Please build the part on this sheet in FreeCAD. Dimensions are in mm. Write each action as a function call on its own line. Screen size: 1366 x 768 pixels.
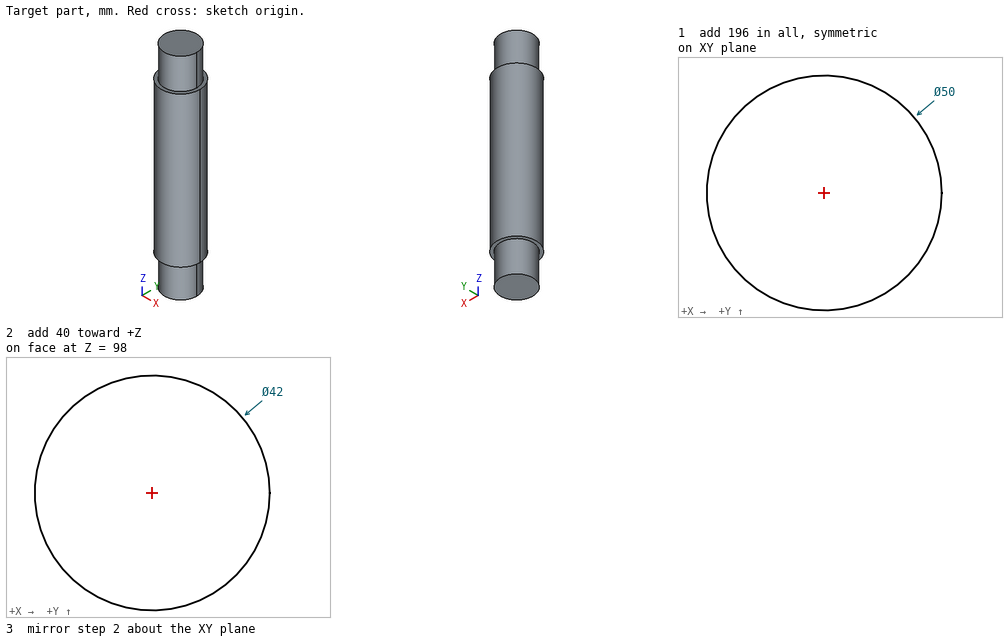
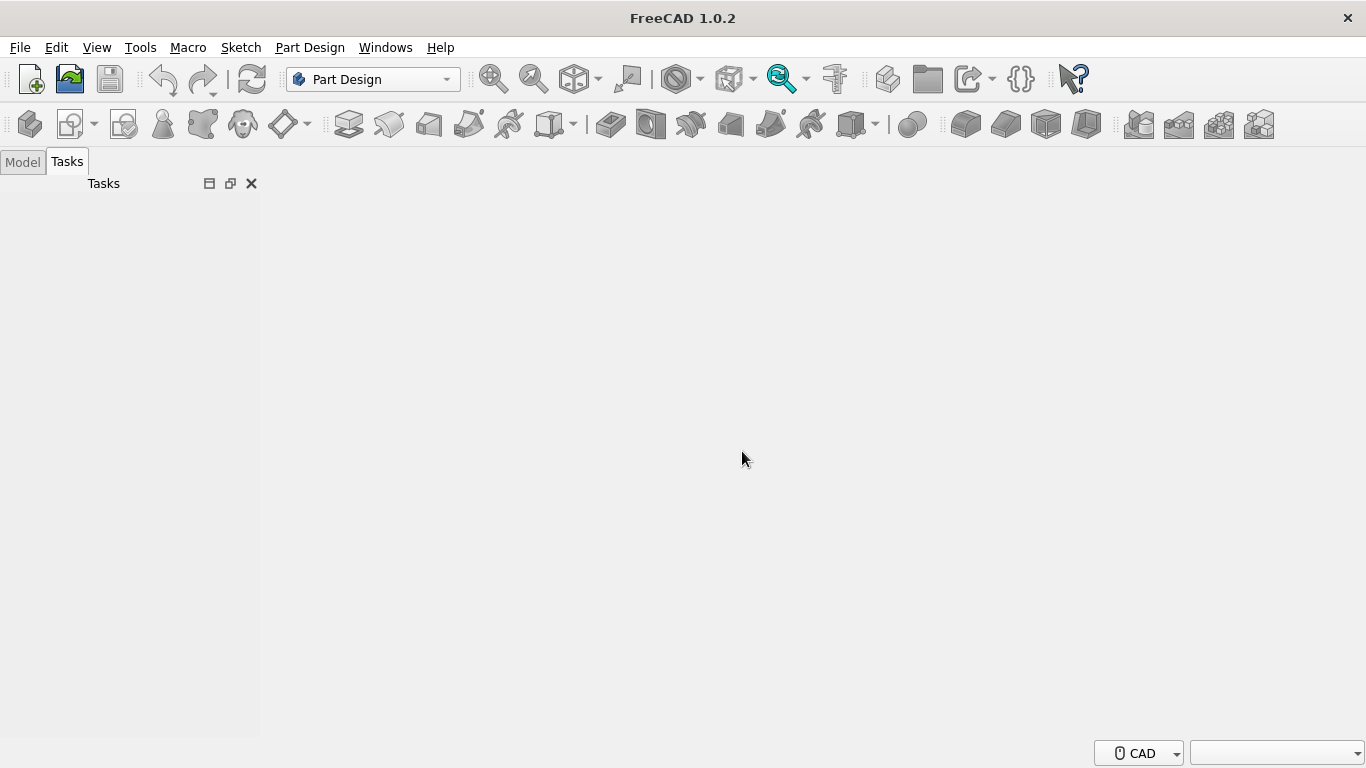
click(30, 80)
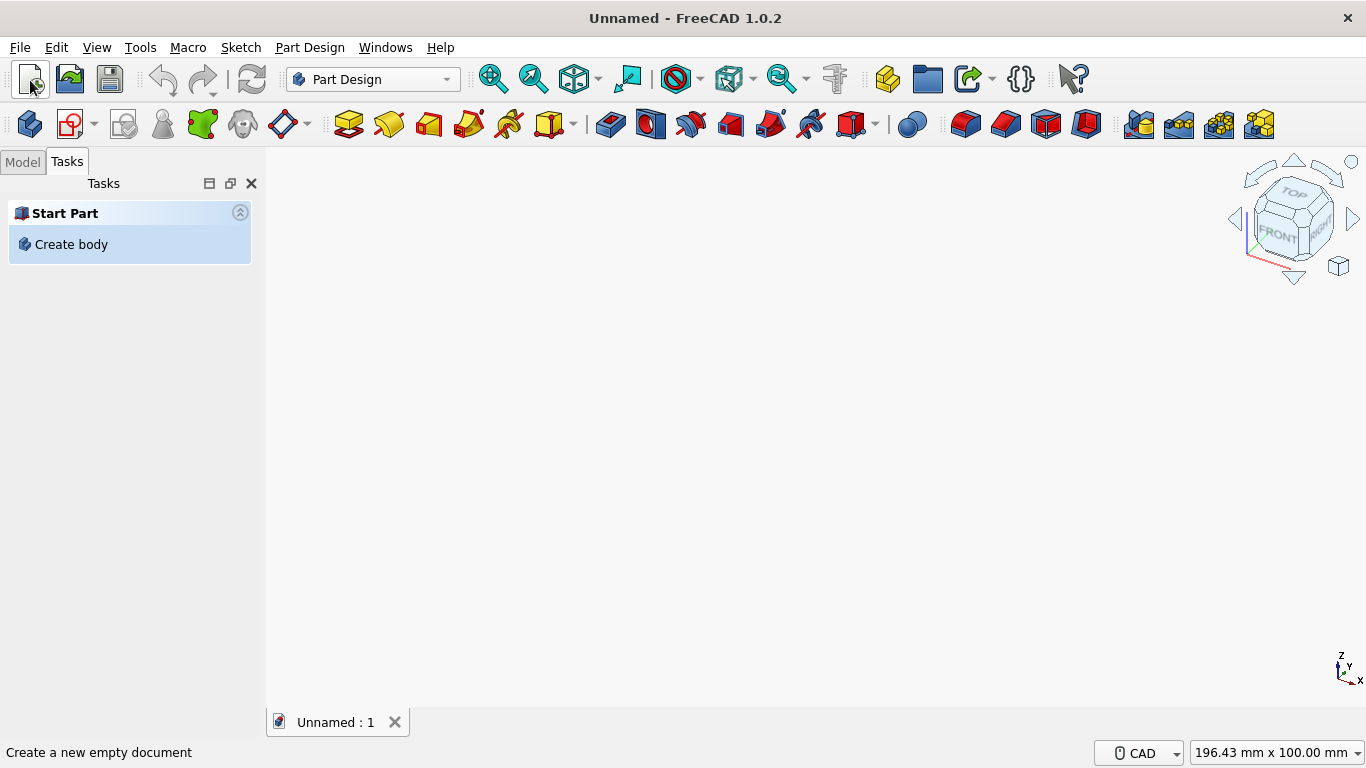
click(70, 124)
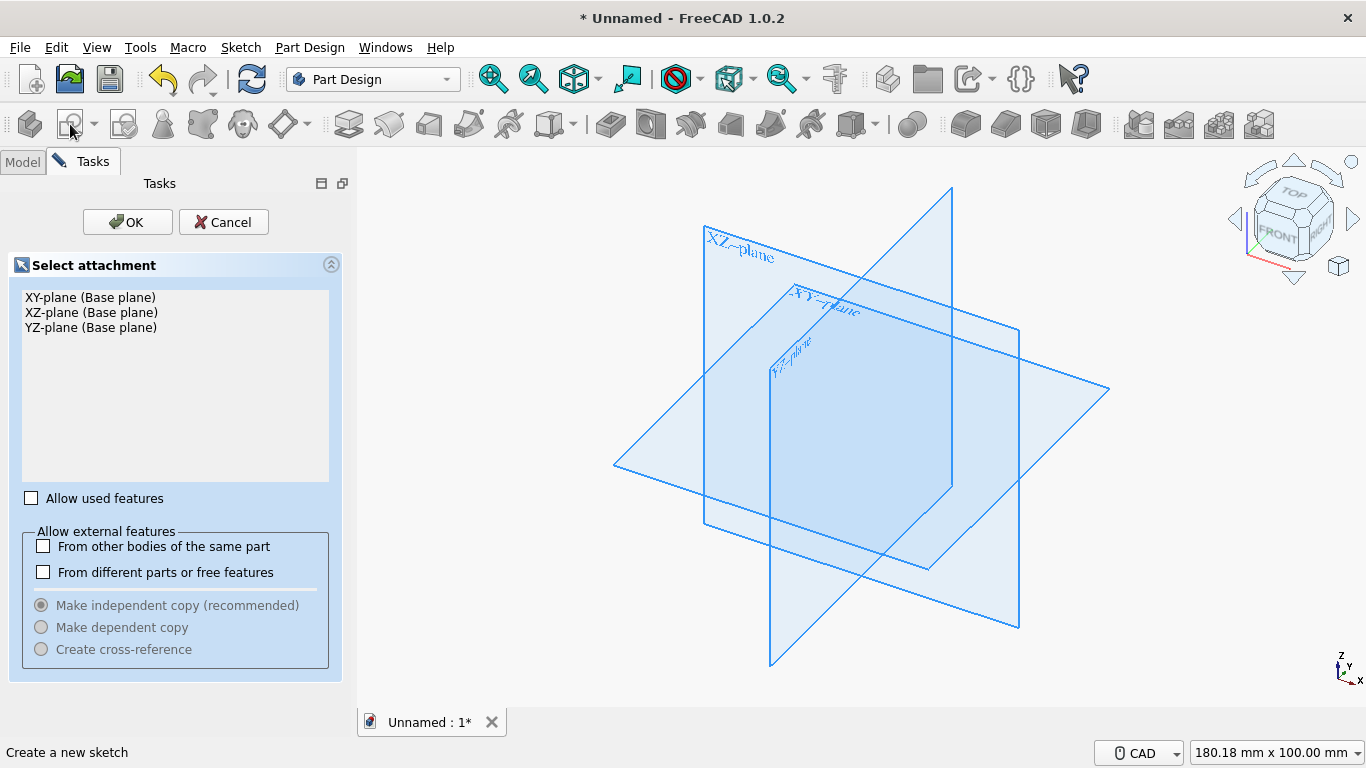
click(82, 298)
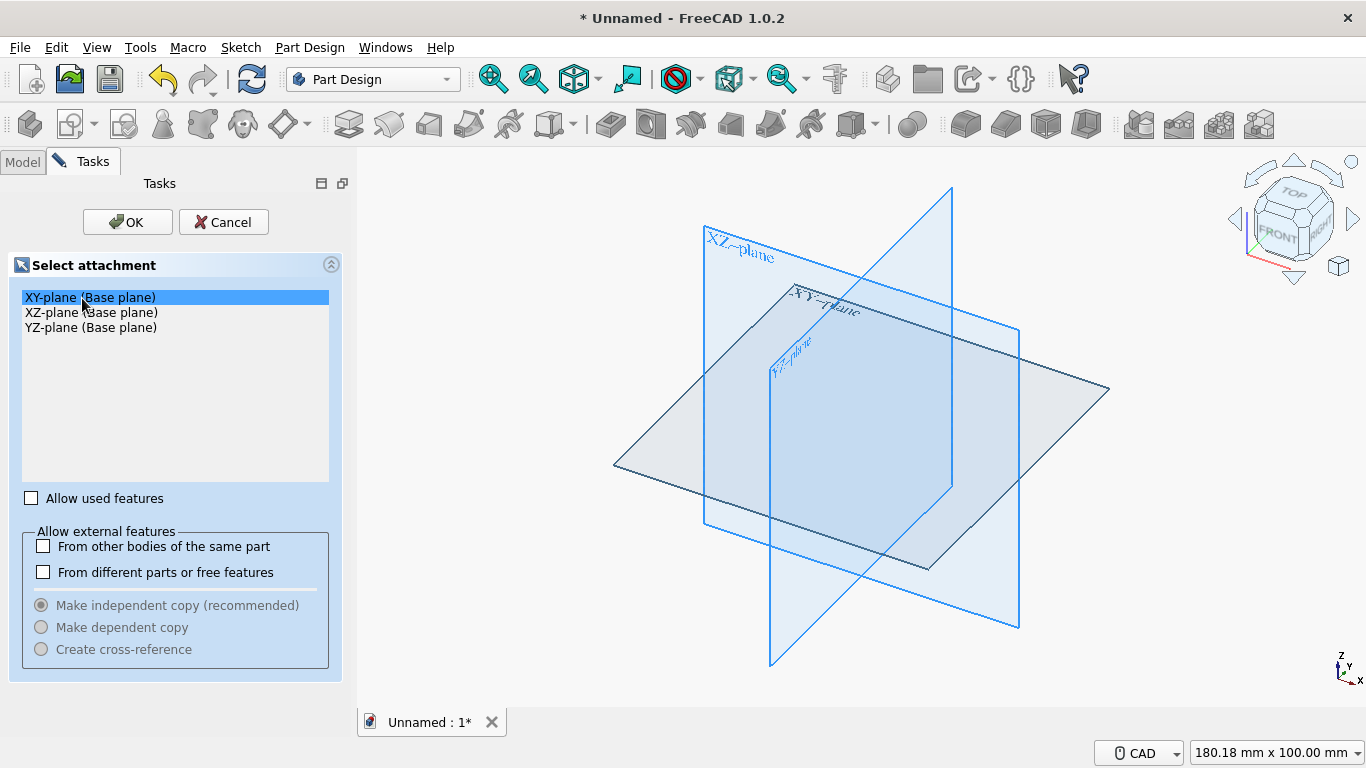
click(128, 222)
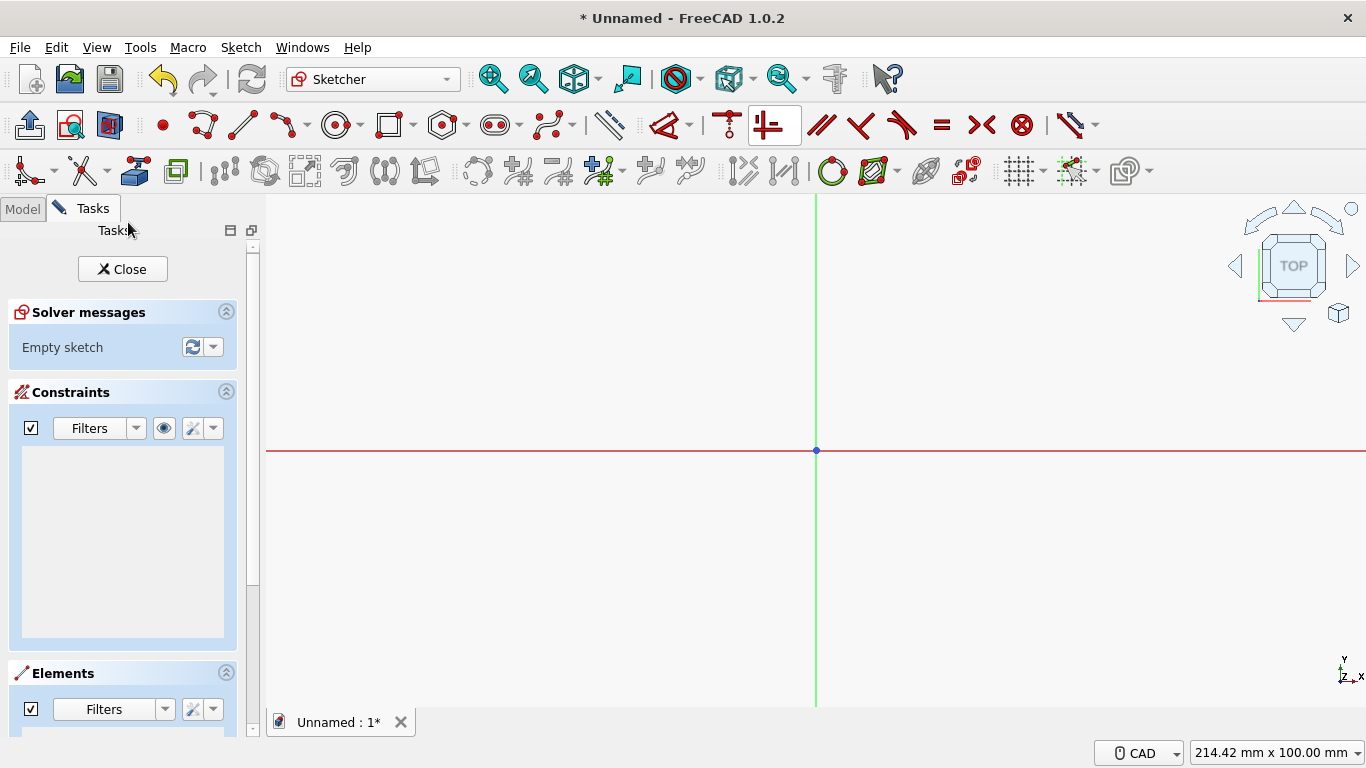
click(336, 126)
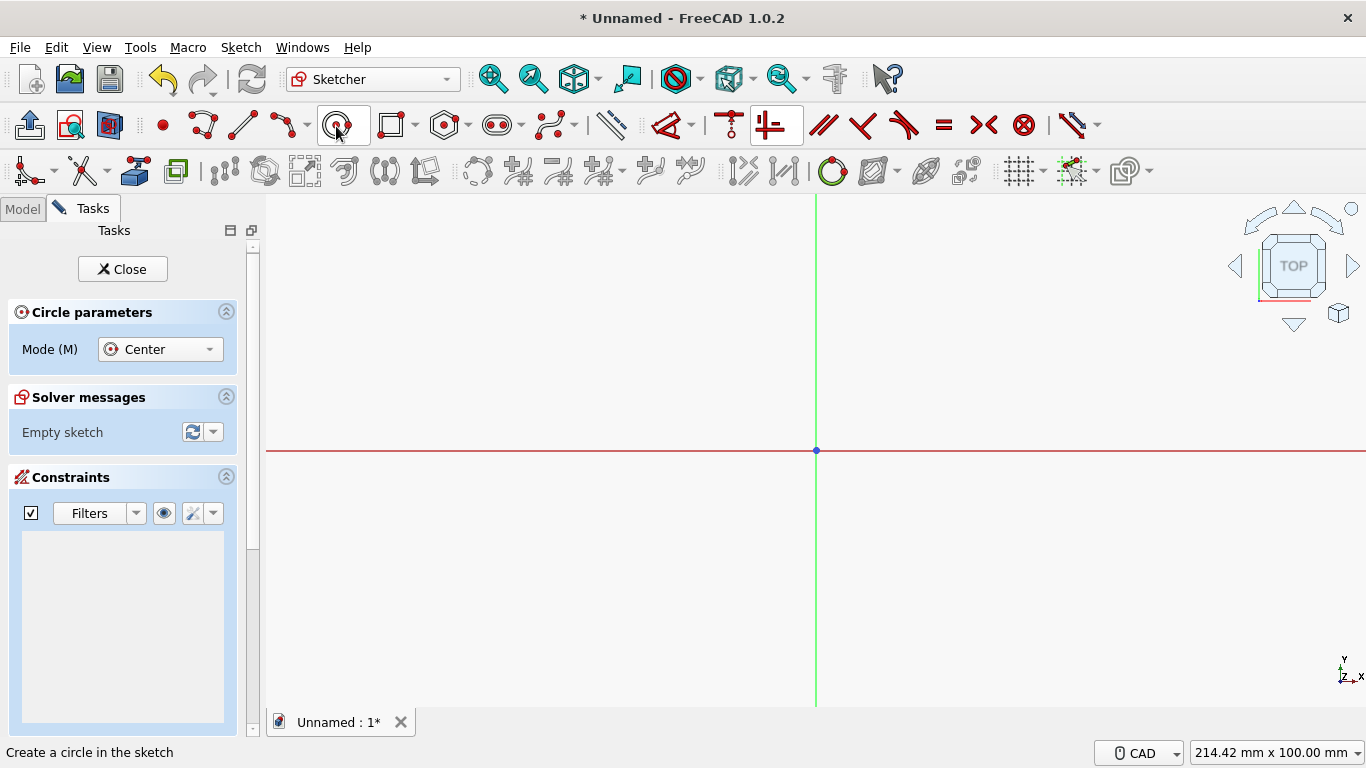
click(816, 450)
move(907, 360)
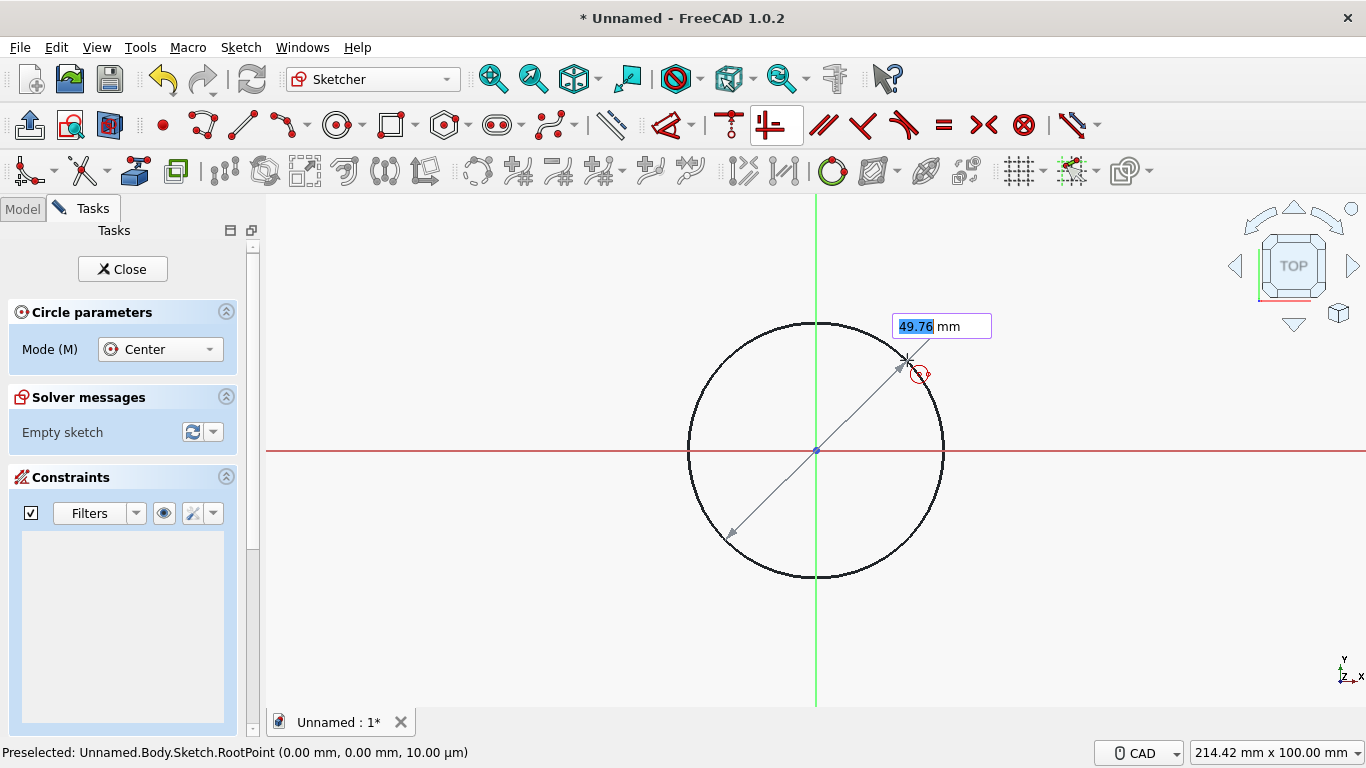
text(50)
key(Return)
key(Escape)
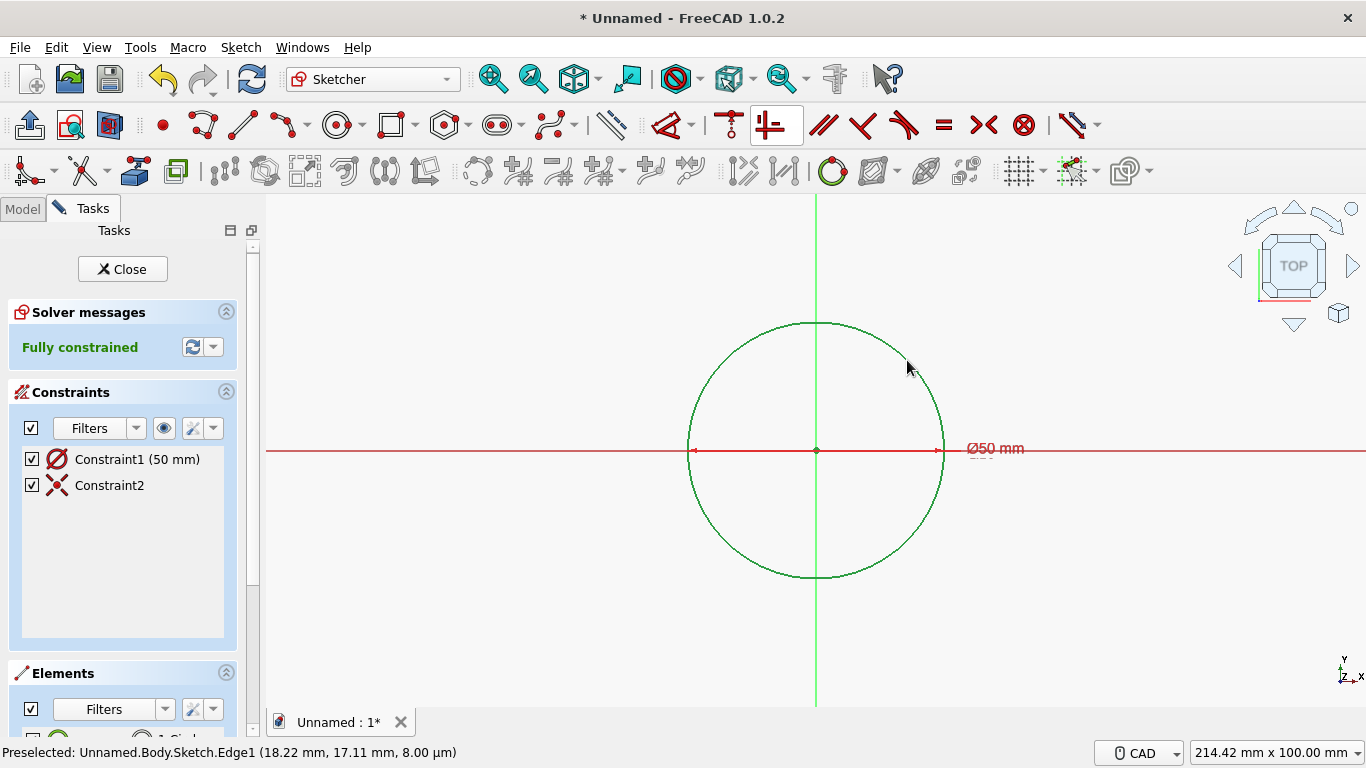
click(123, 269)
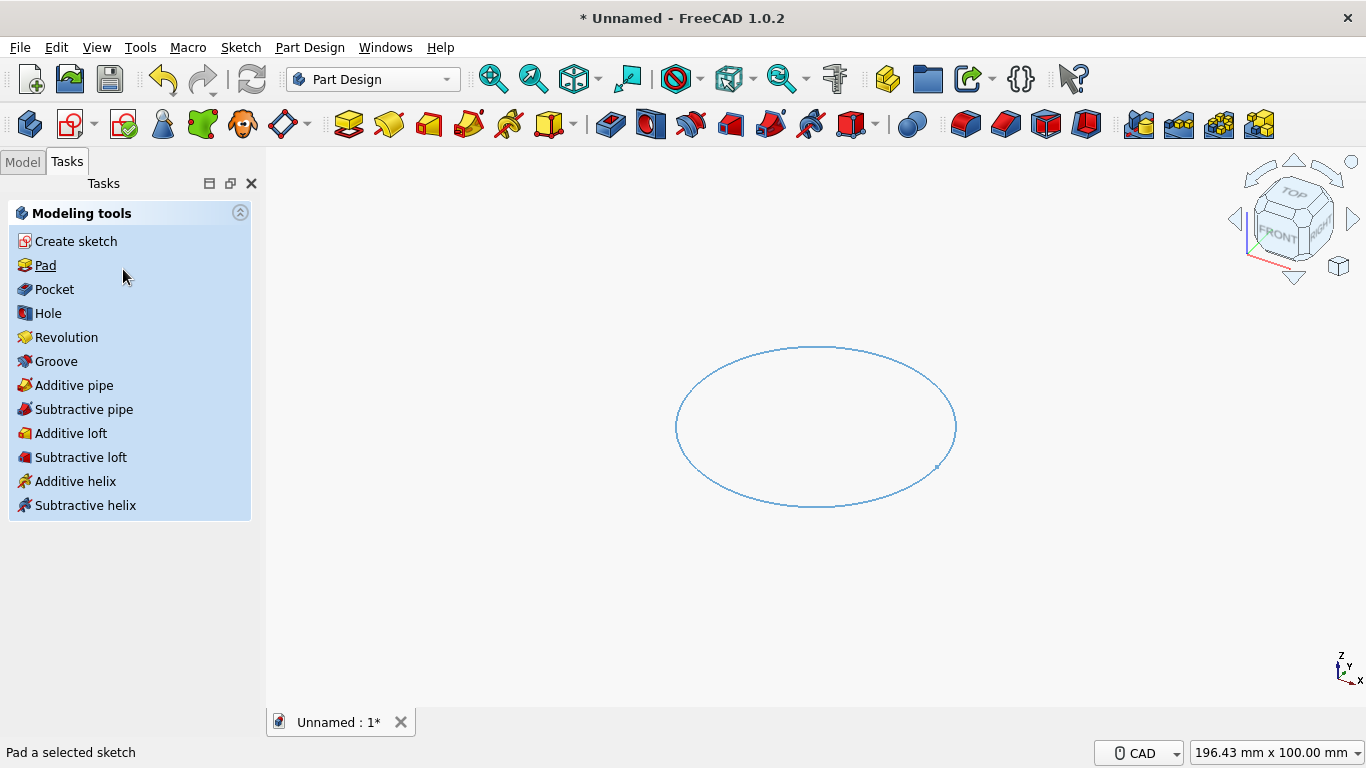
click(350, 124)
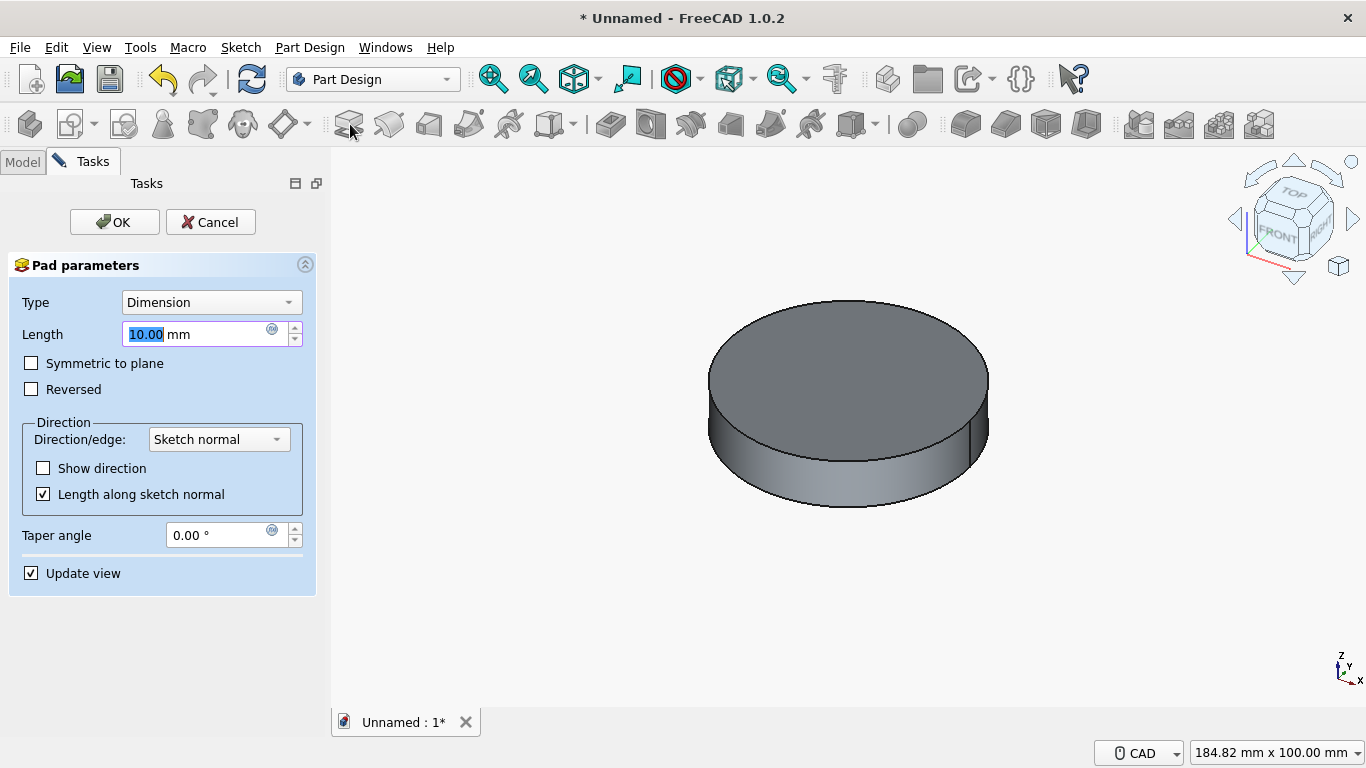
text(196)
key(Tab)